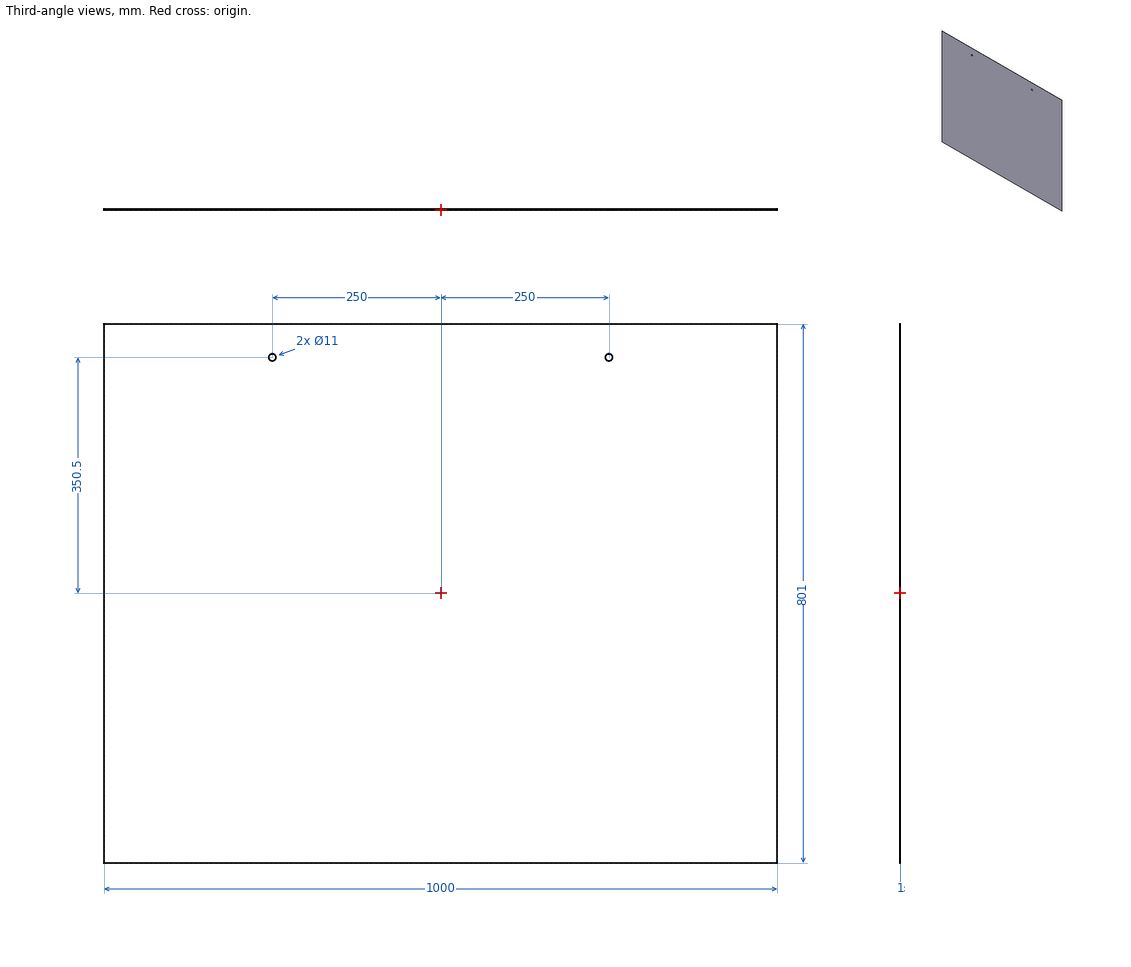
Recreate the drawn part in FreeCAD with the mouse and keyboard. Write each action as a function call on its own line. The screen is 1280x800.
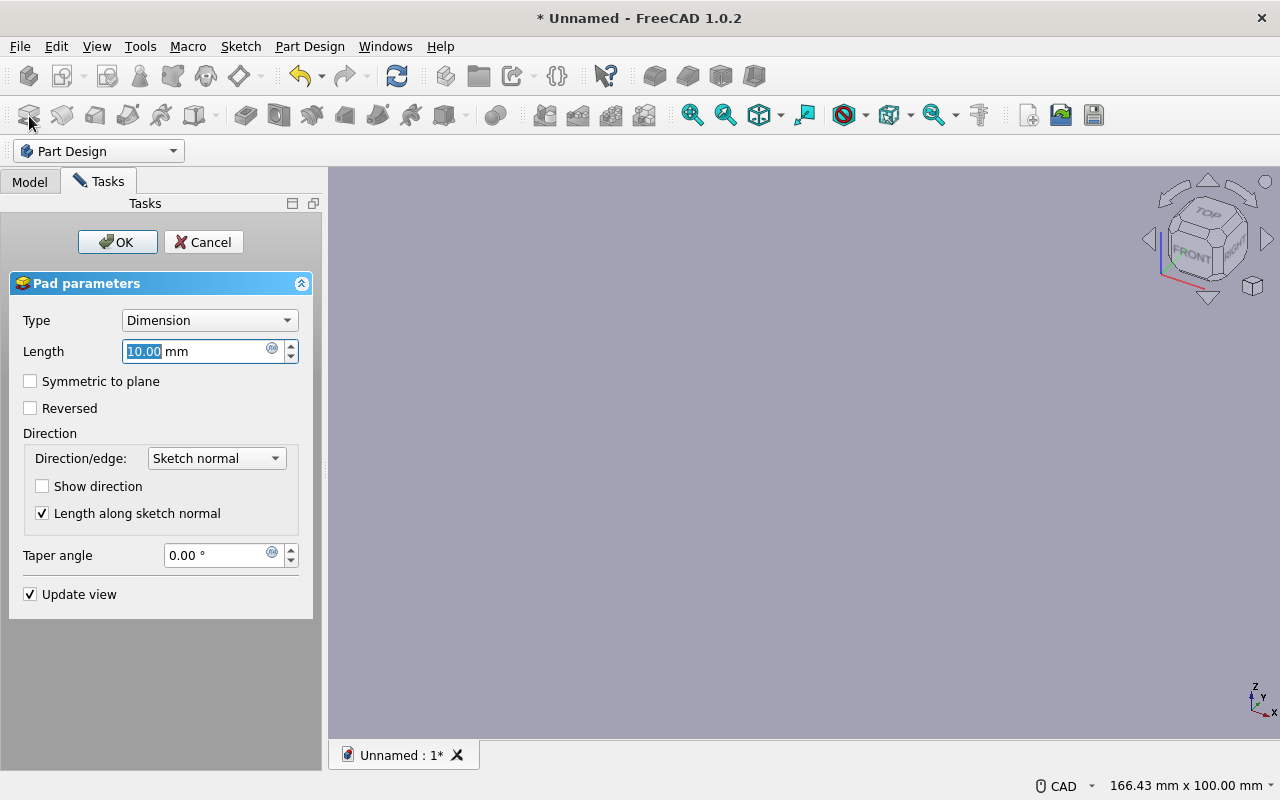
text(1)
key(Tab)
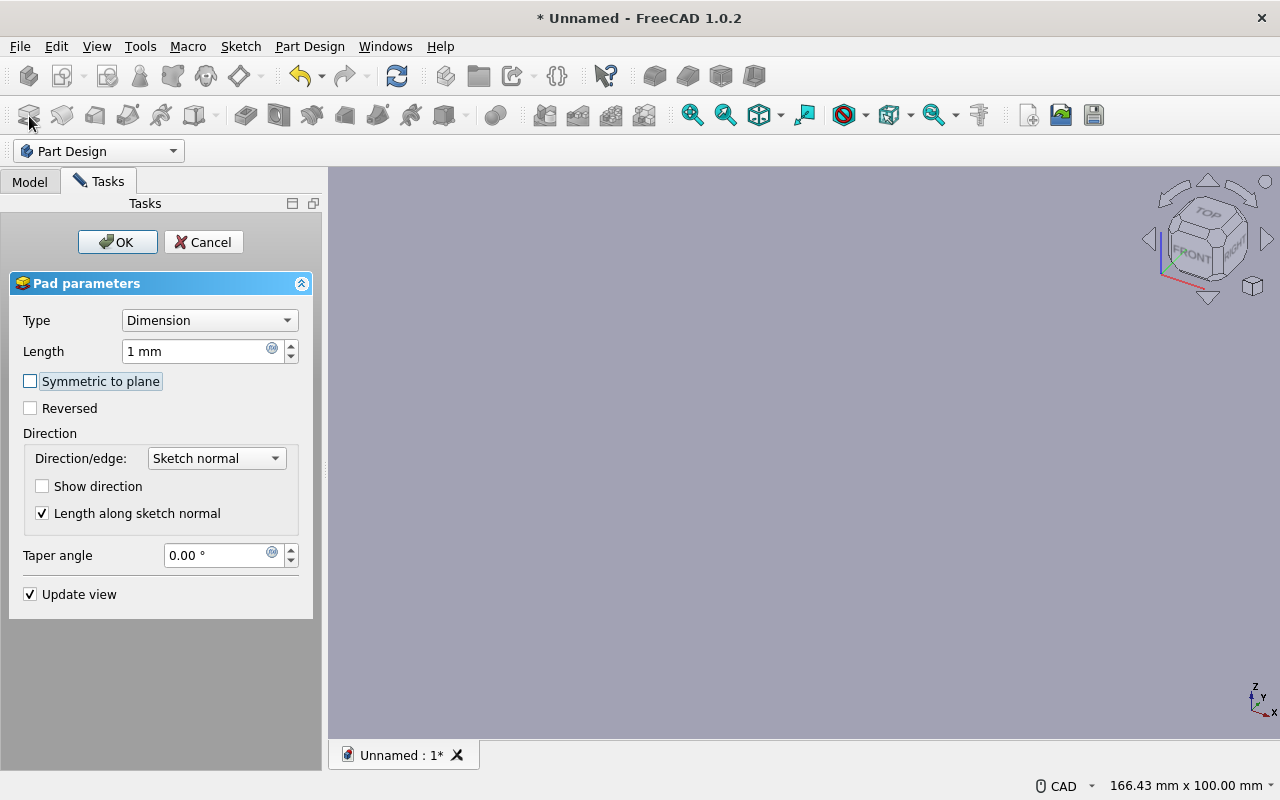
click(31, 408)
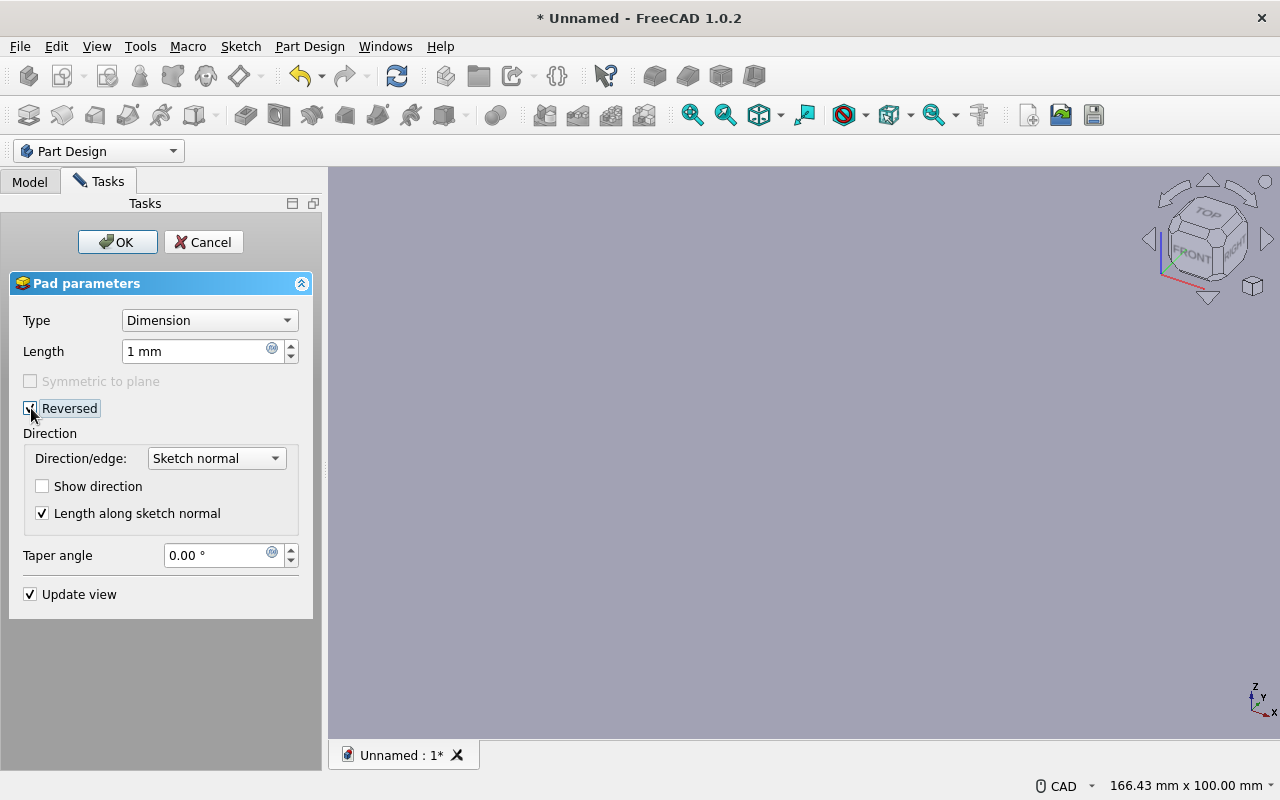
click(118, 242)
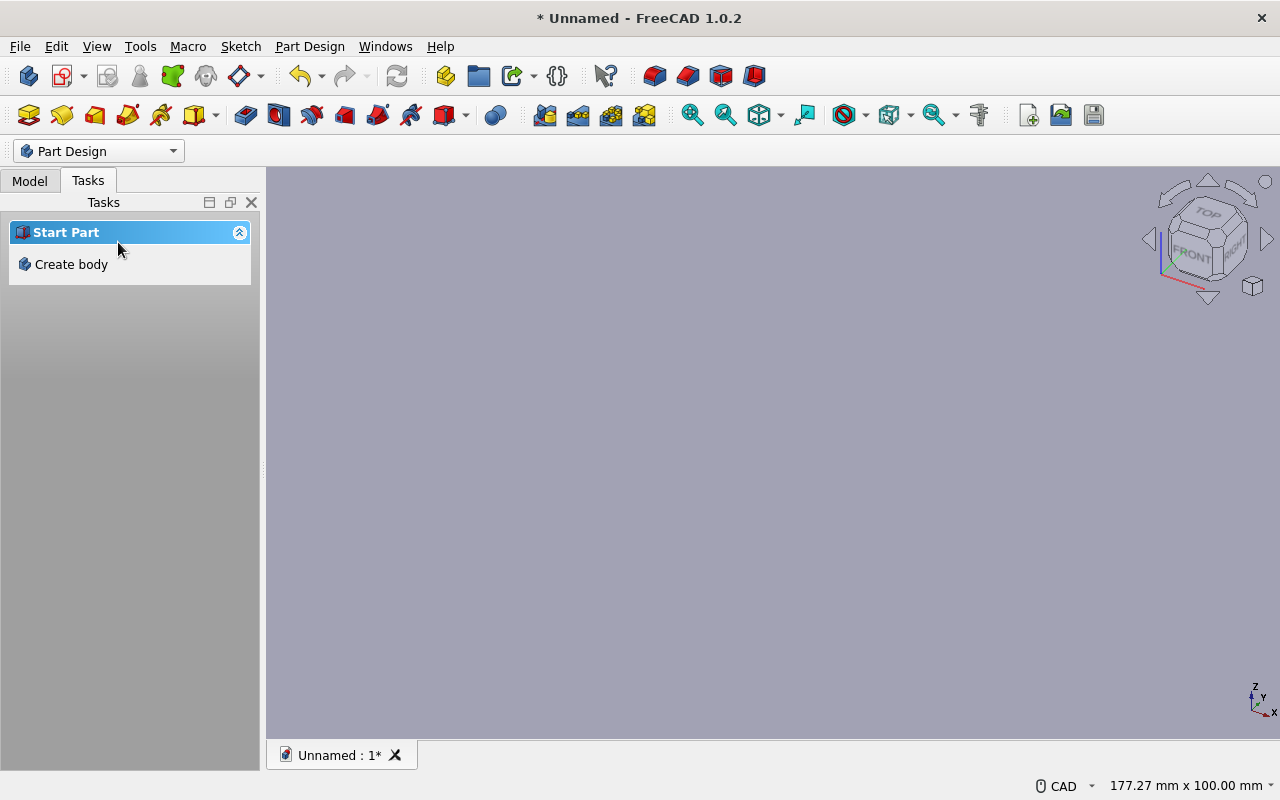
click(693, 116)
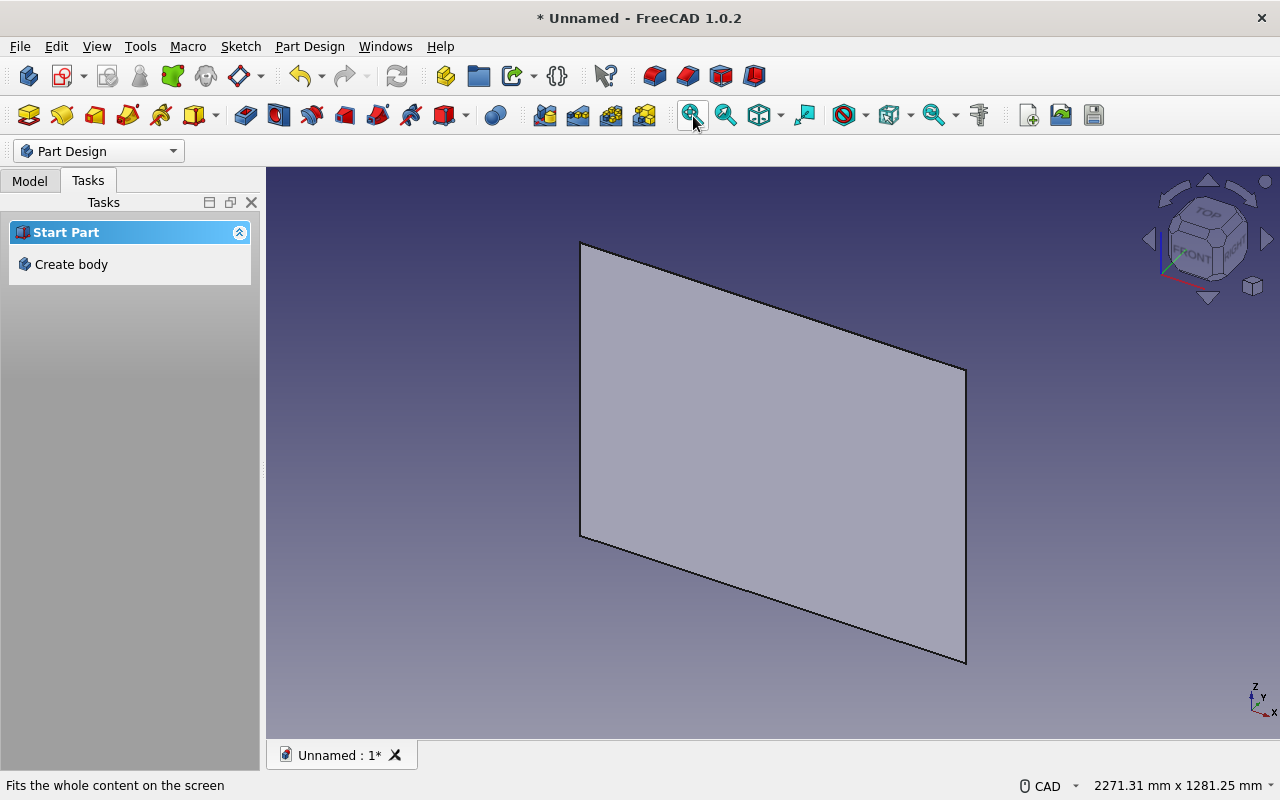
key(4)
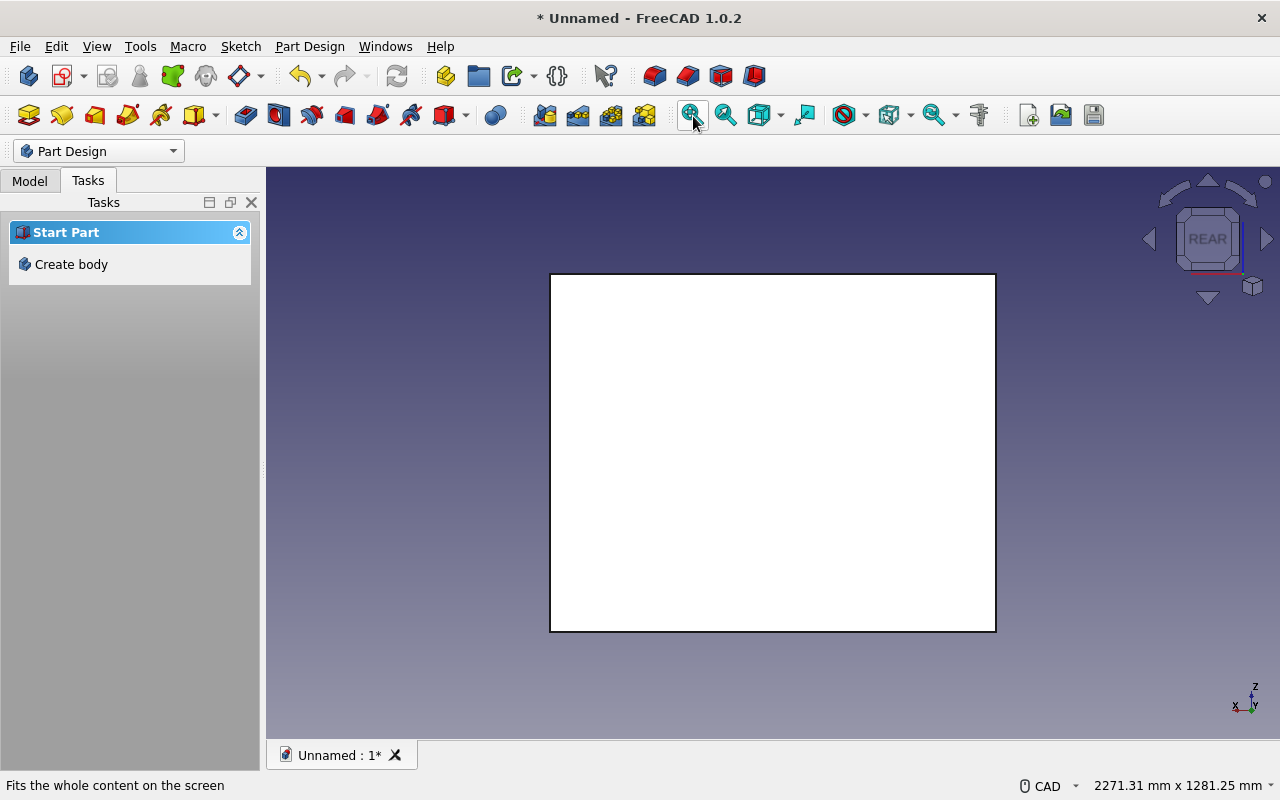
click(773, 452)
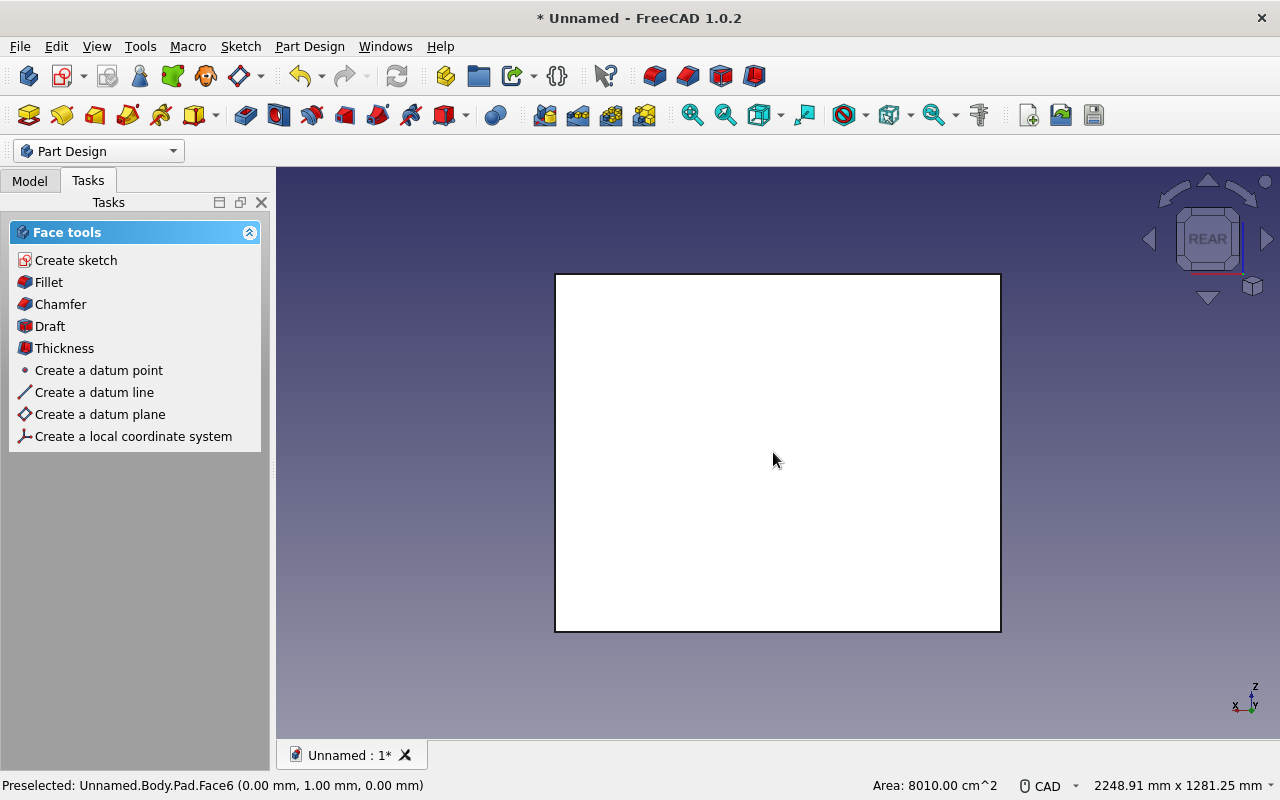
click(62, 76)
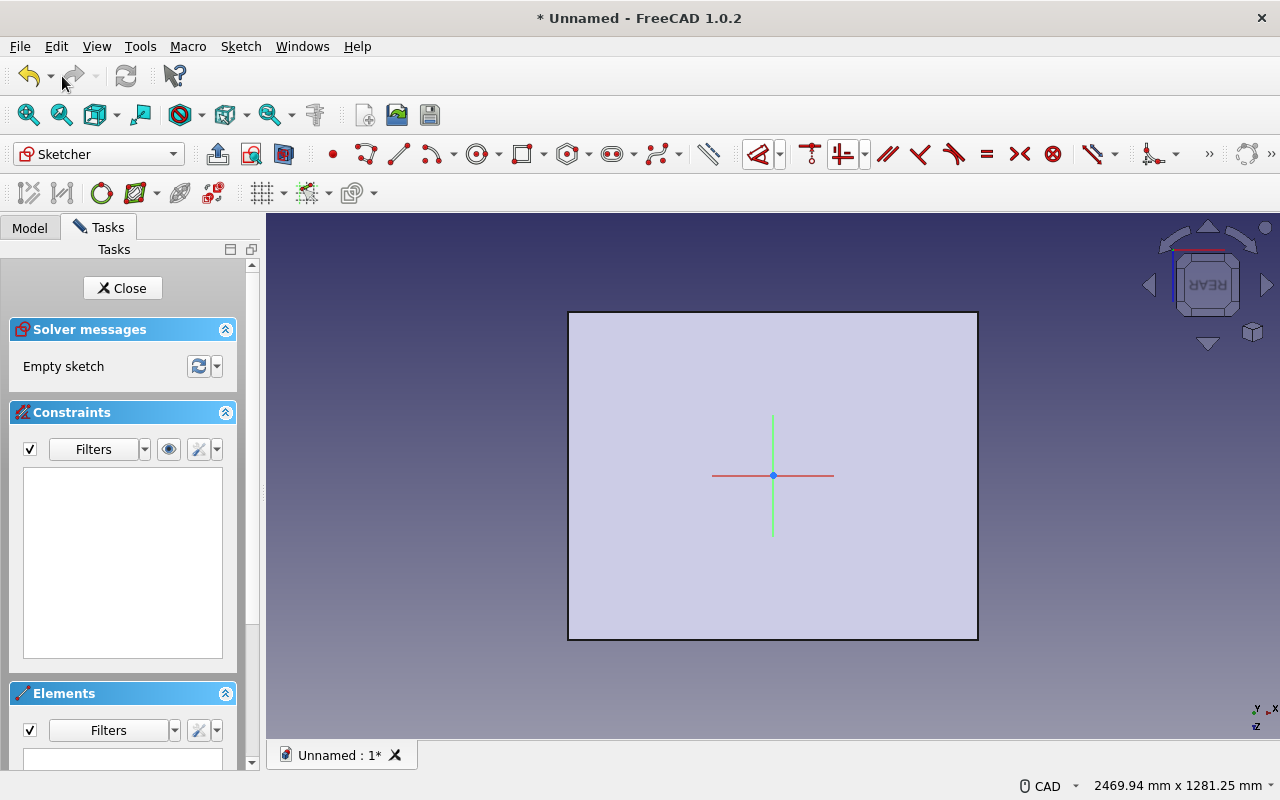
scroll(829, 609, up, 4)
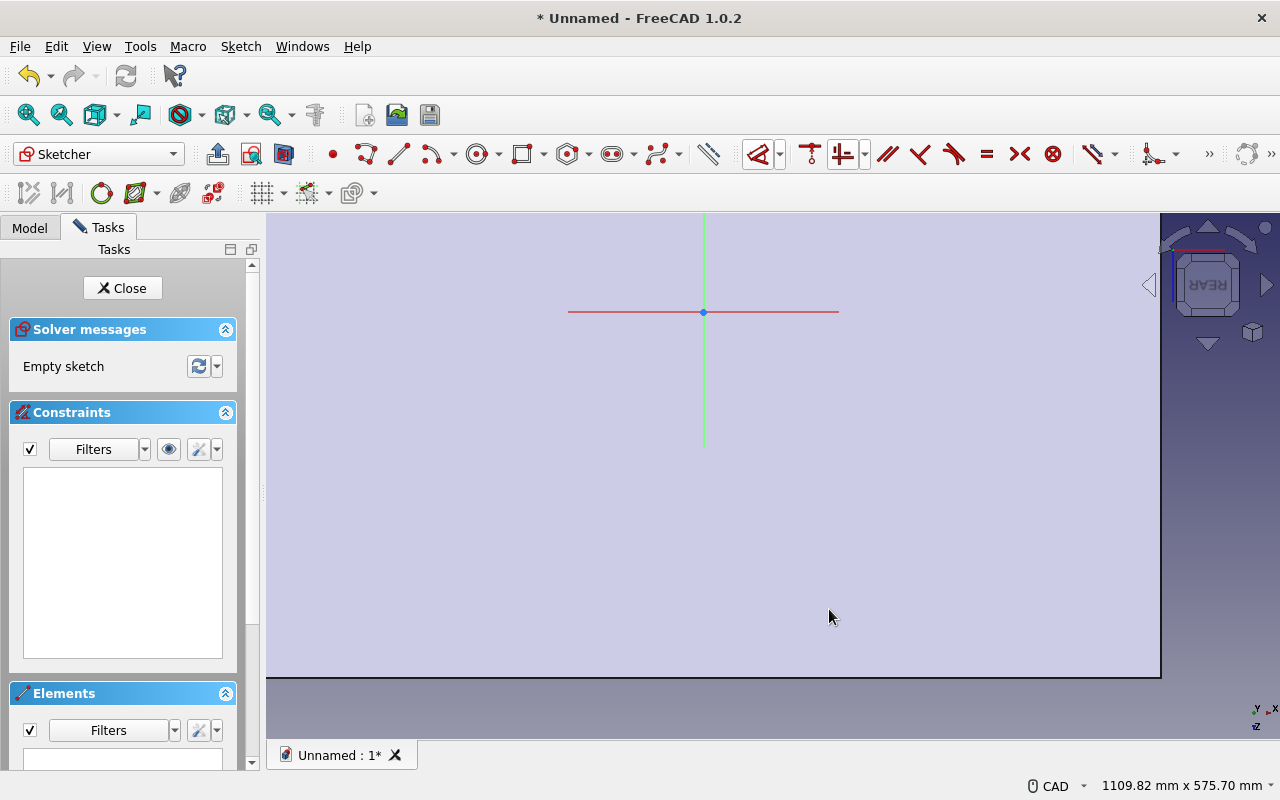
click(476, 154)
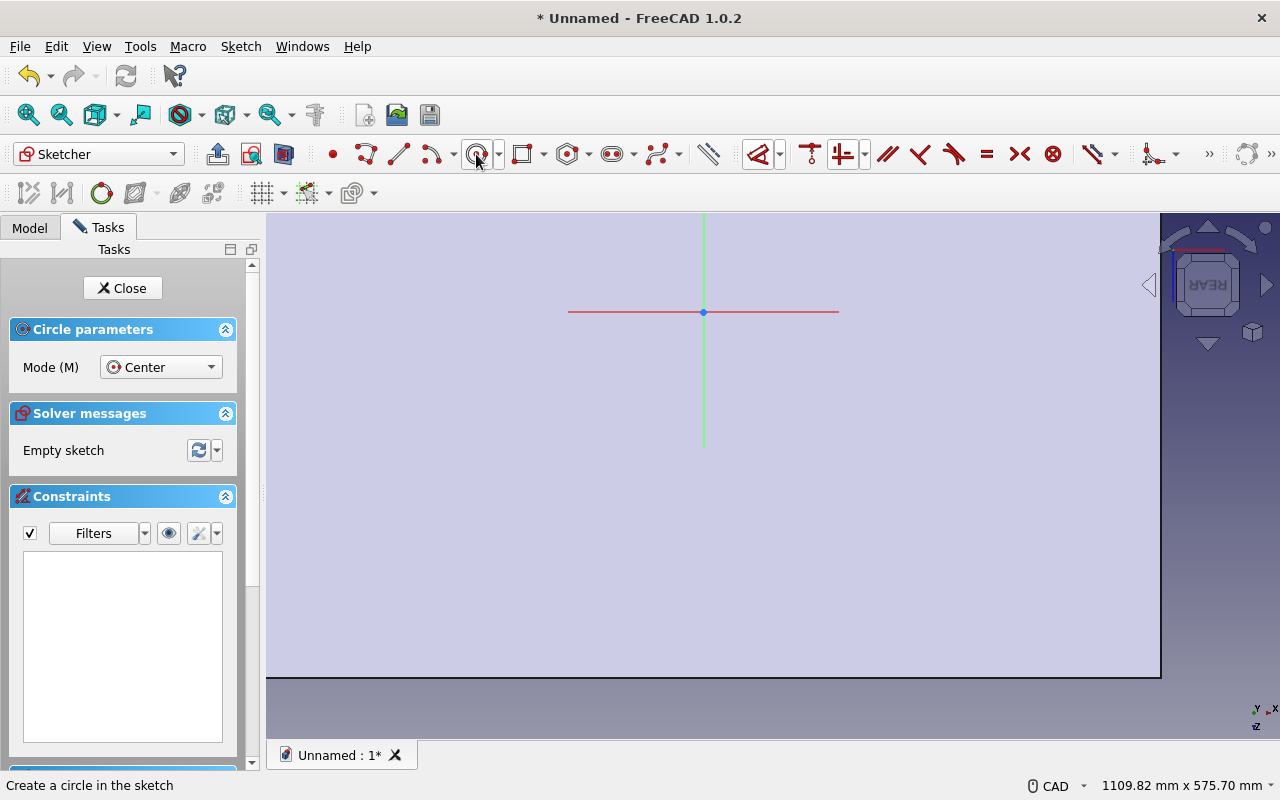
scroll(475, 632, up, 8)